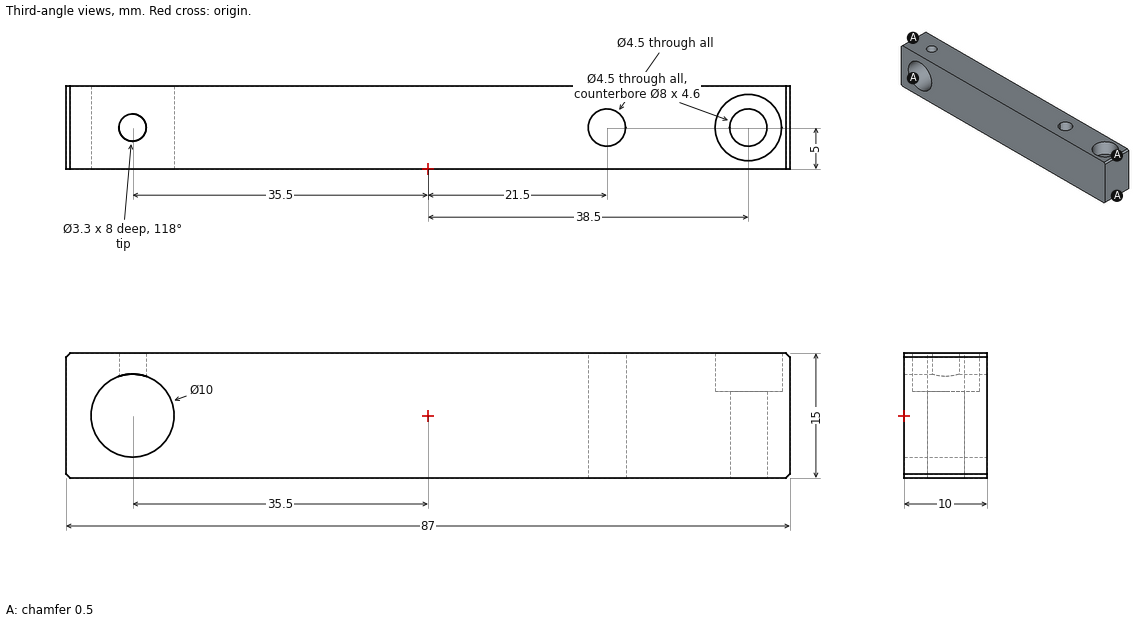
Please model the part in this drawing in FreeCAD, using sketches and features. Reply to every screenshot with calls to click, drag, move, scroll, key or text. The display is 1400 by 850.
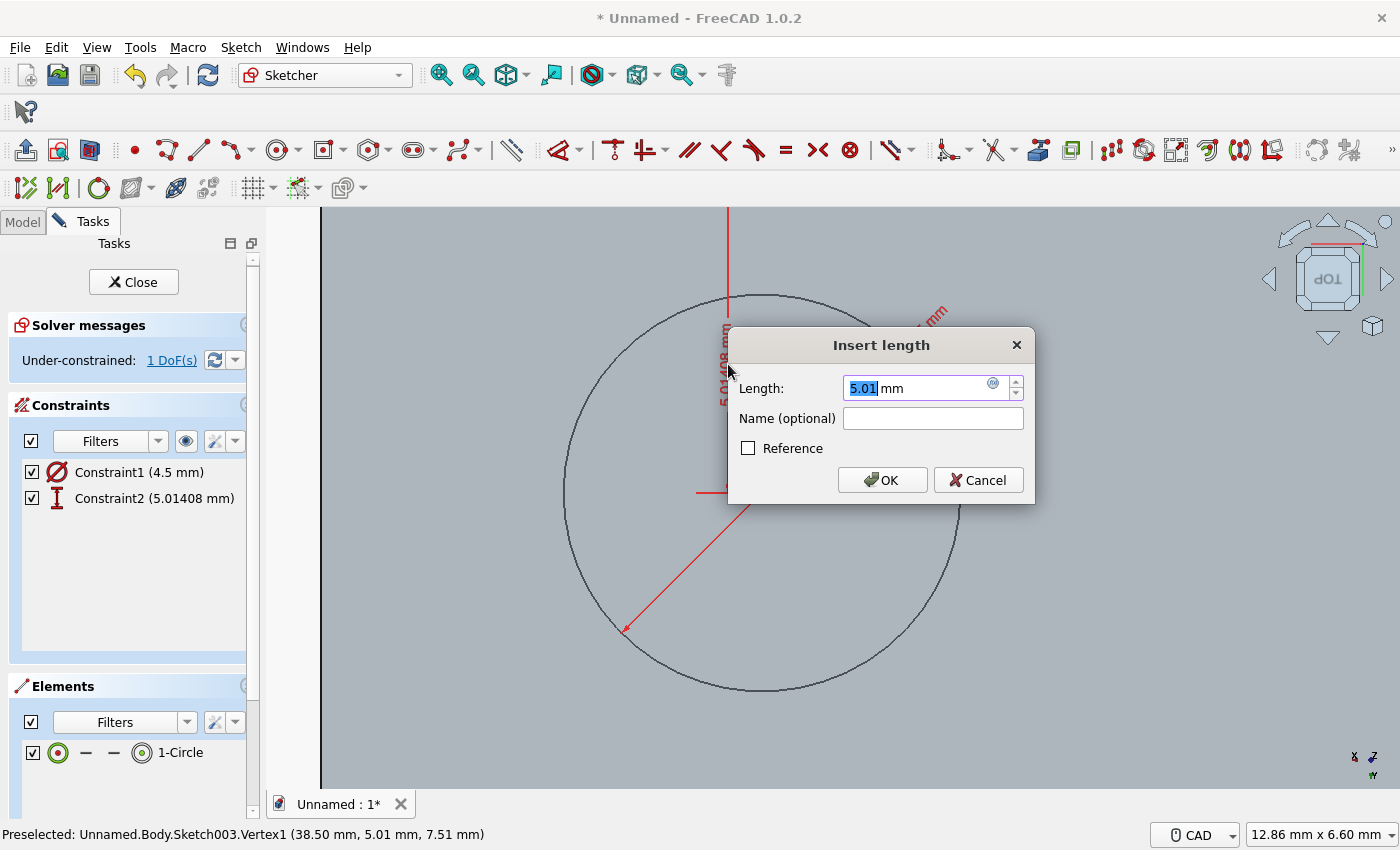
text(5)
key(Return)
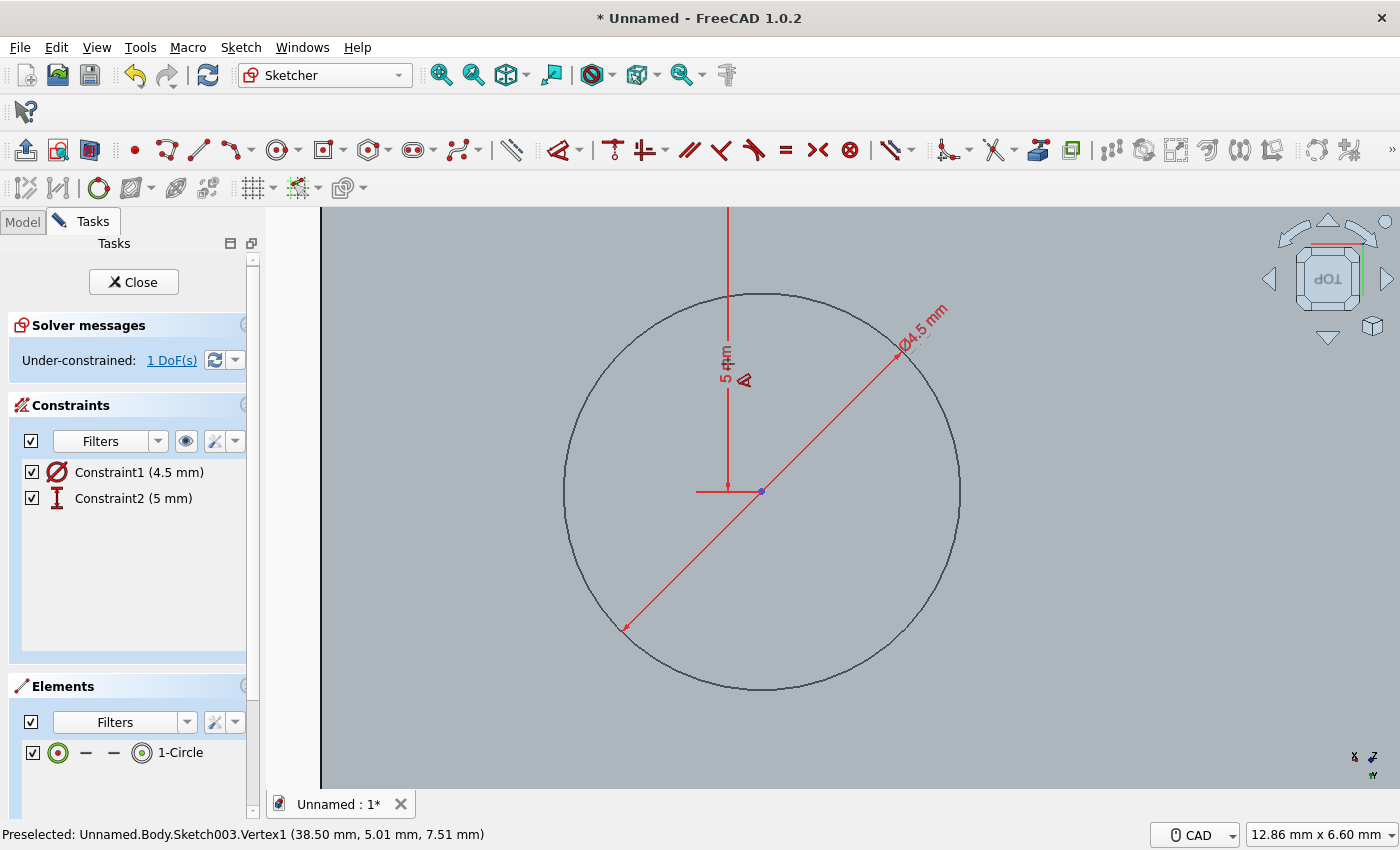
click(762, 492)
click(998, 526)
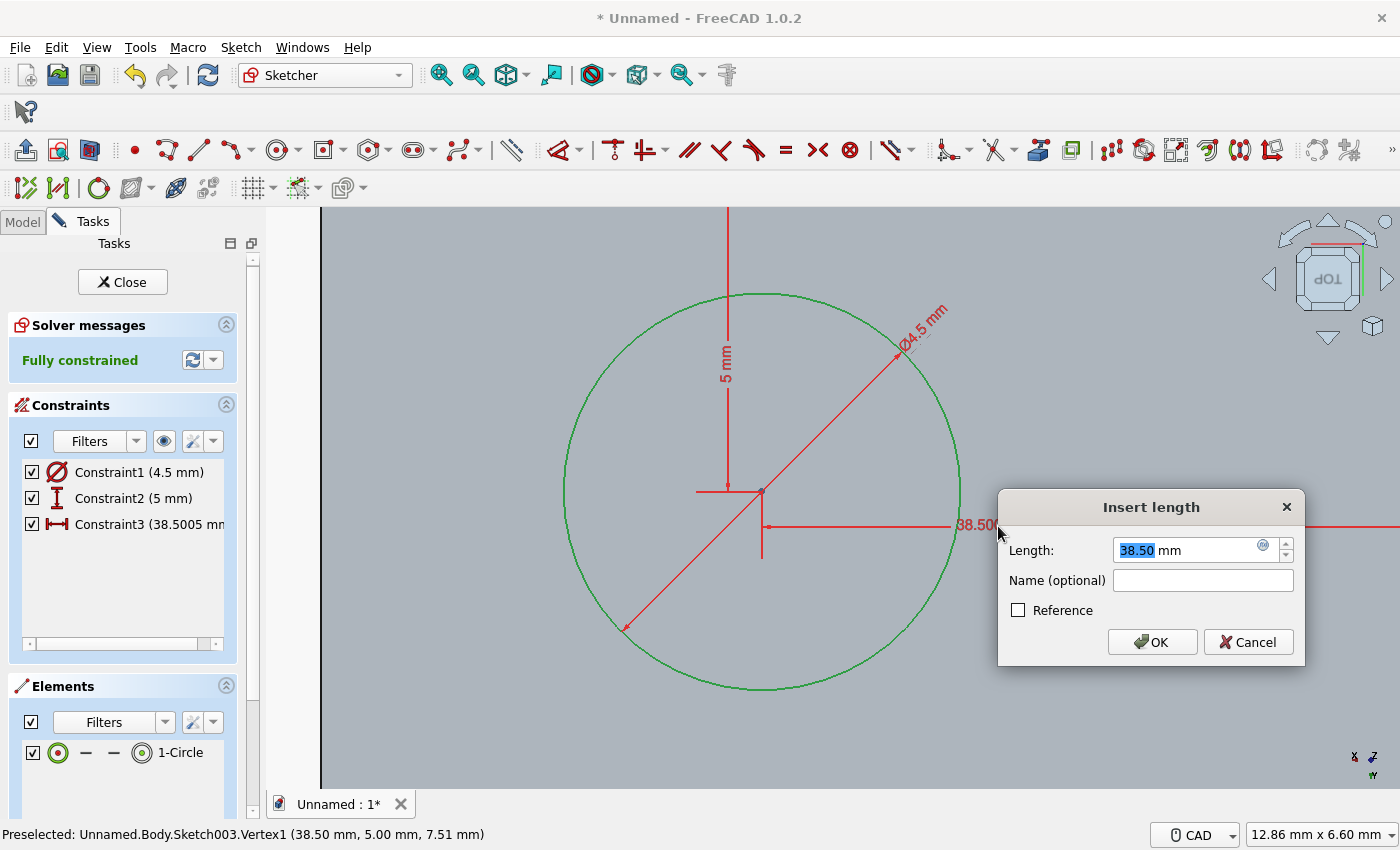
text(38.5)
key(Return)
key(Escape)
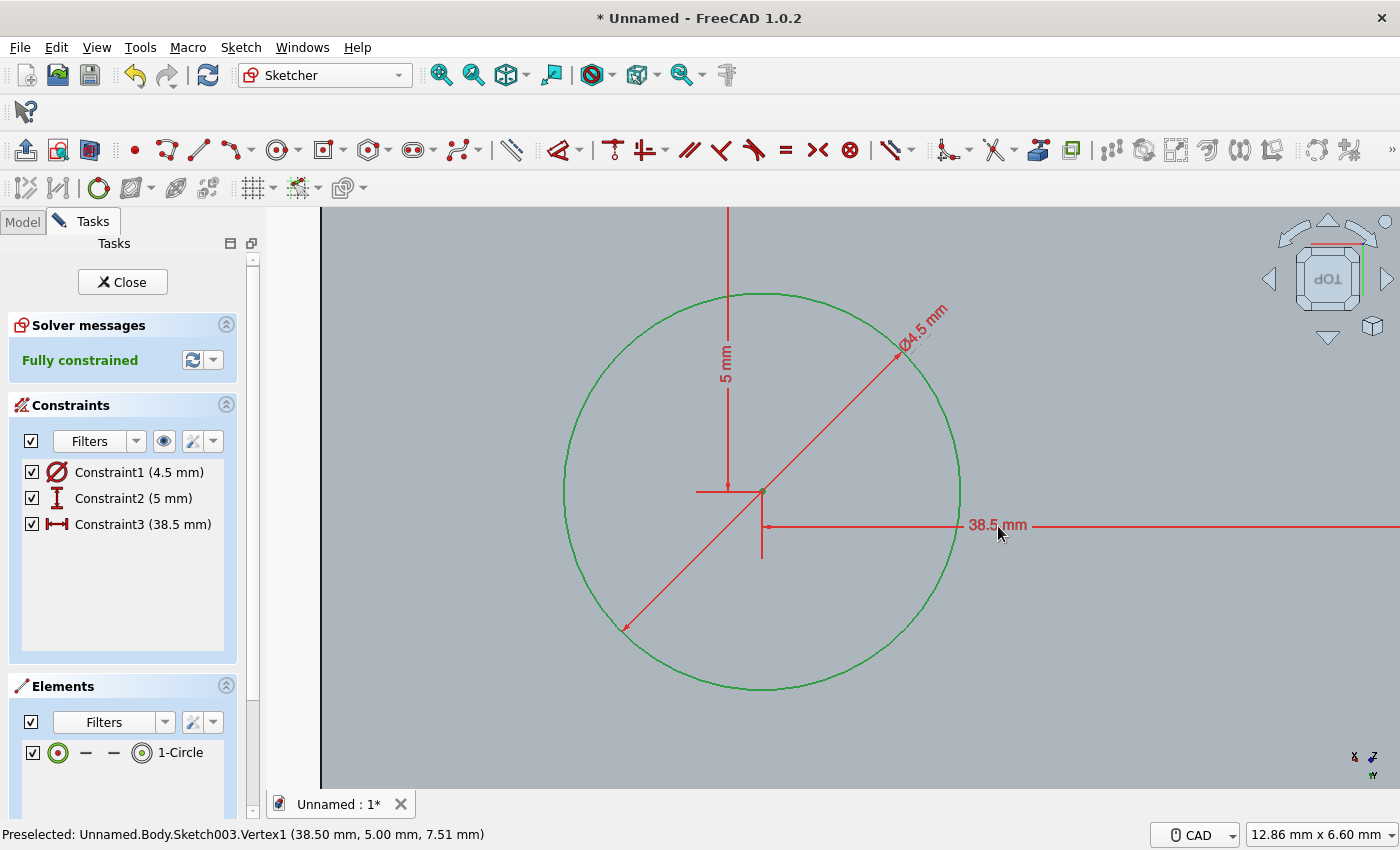
click(123, 282)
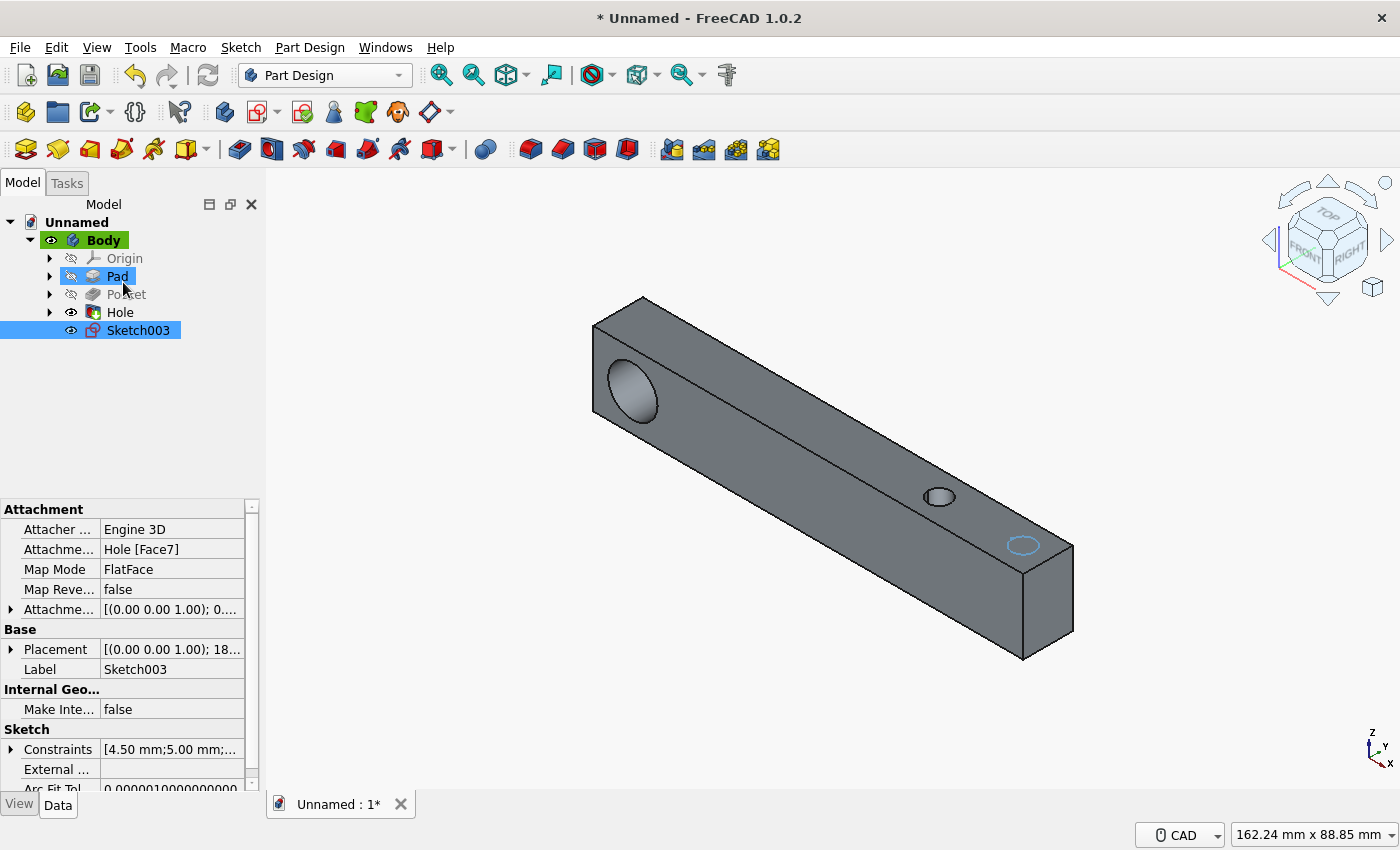
click(272, 150)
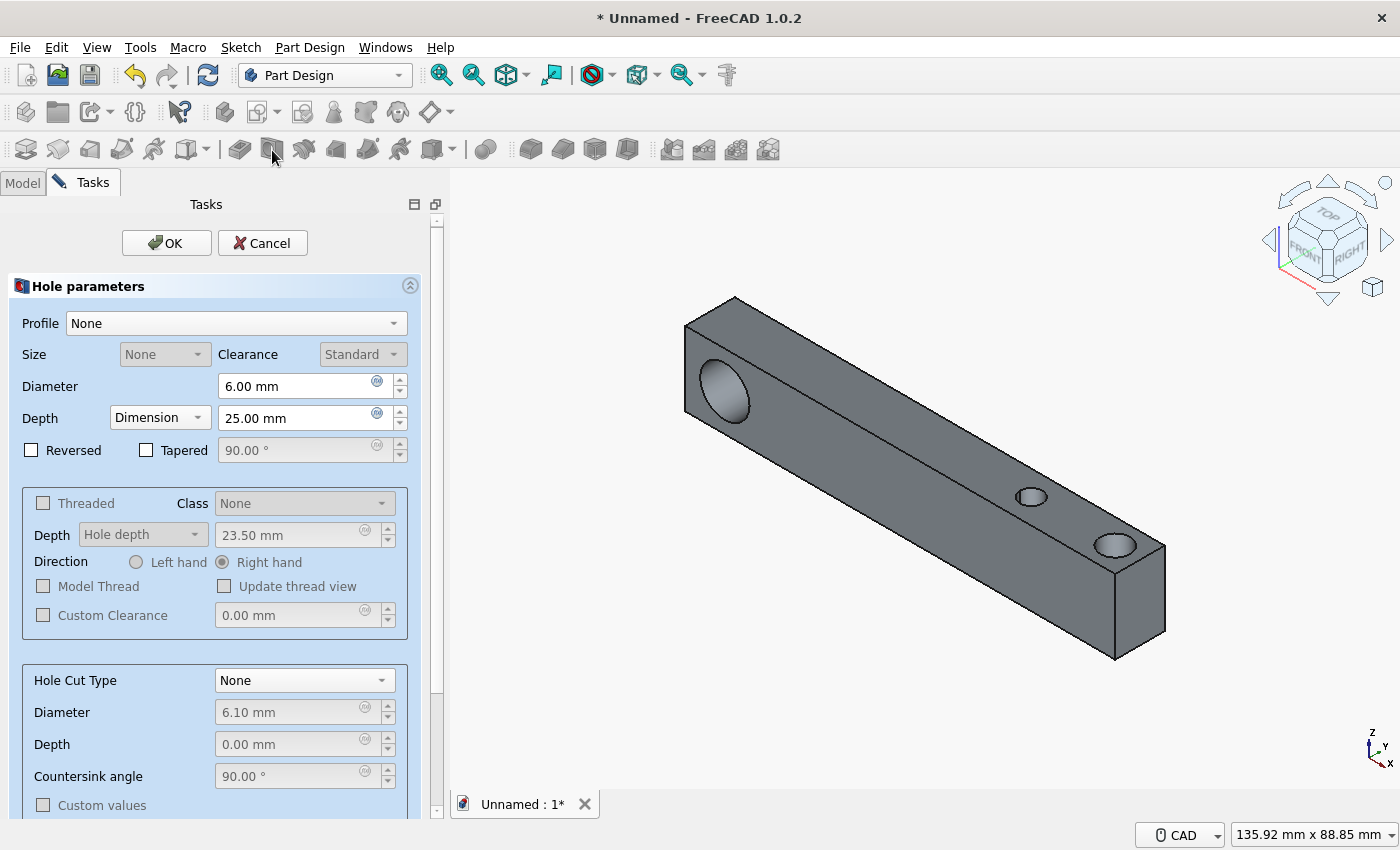
triple_click(305, 386)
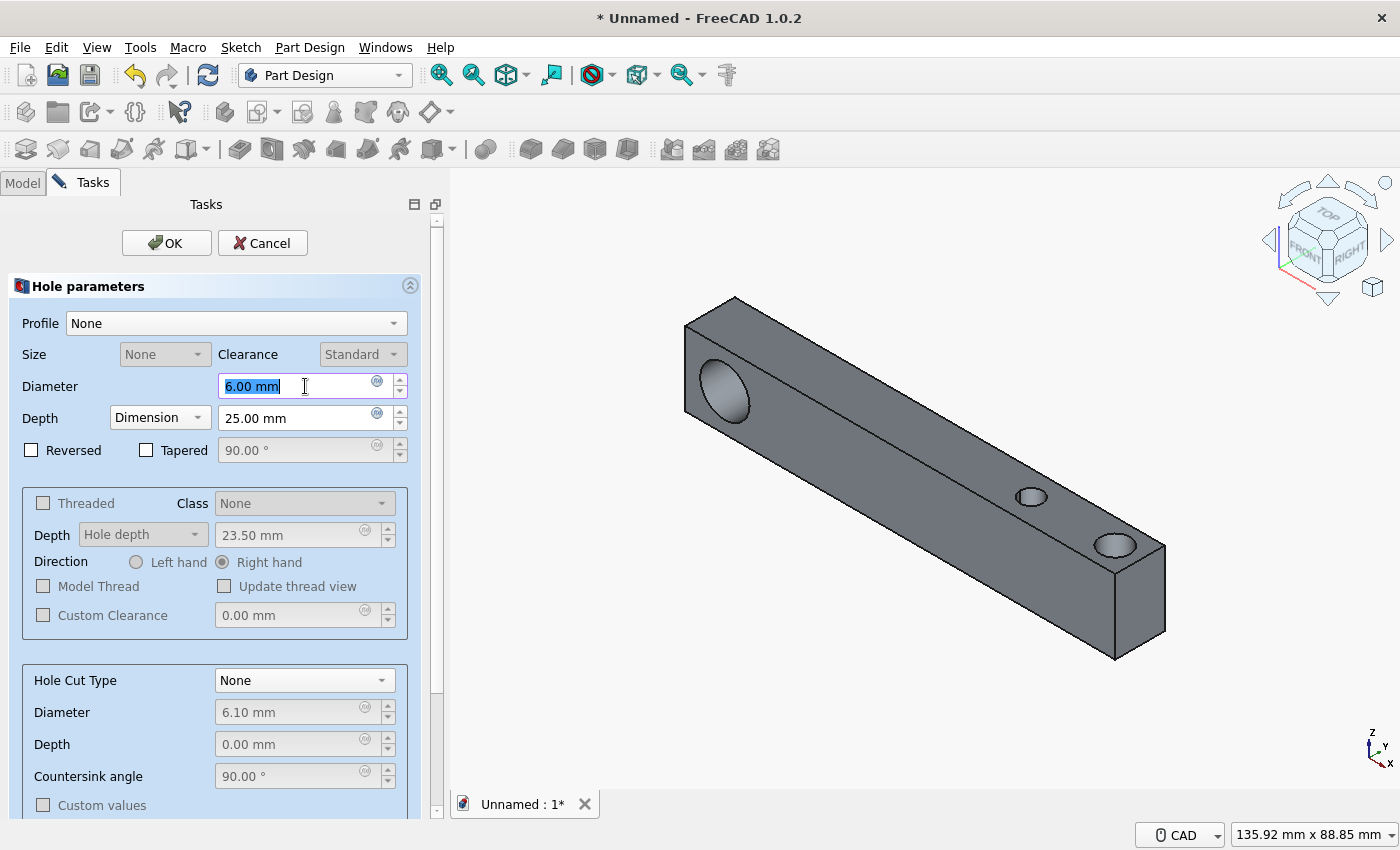
text(4.5)
key(Tab)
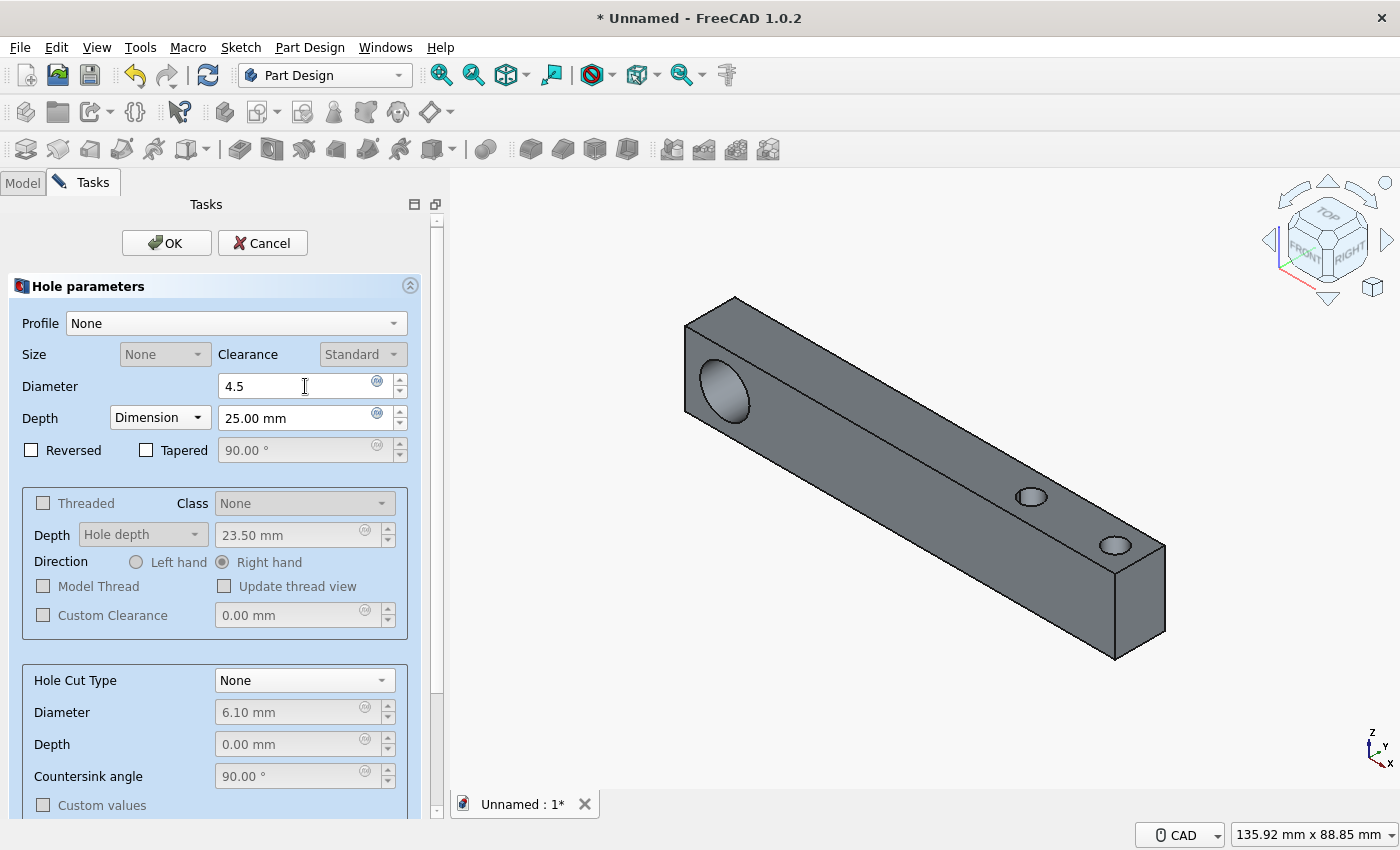
click(161, 418)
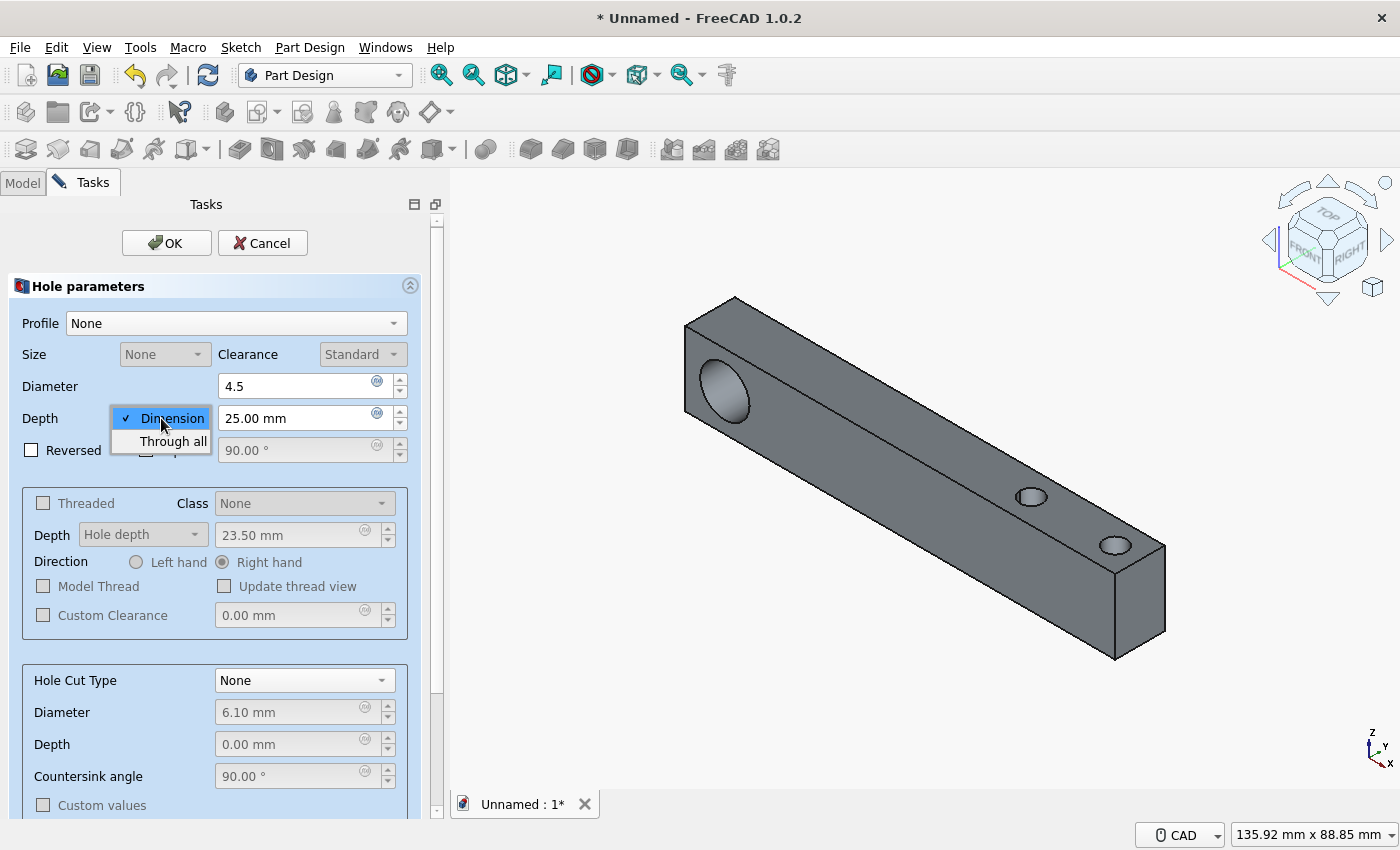
click(160, 442)